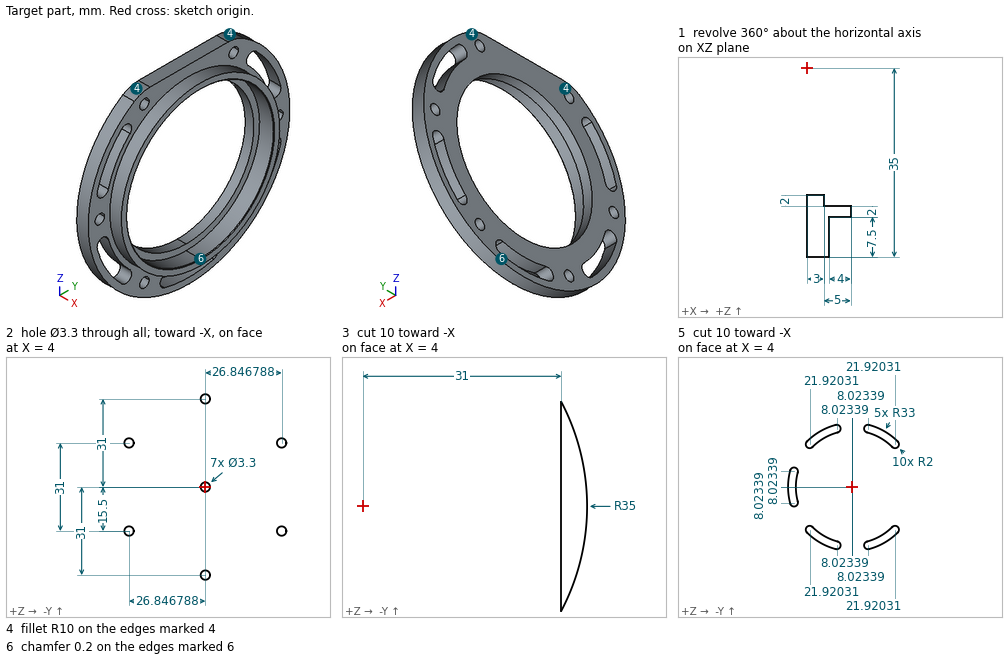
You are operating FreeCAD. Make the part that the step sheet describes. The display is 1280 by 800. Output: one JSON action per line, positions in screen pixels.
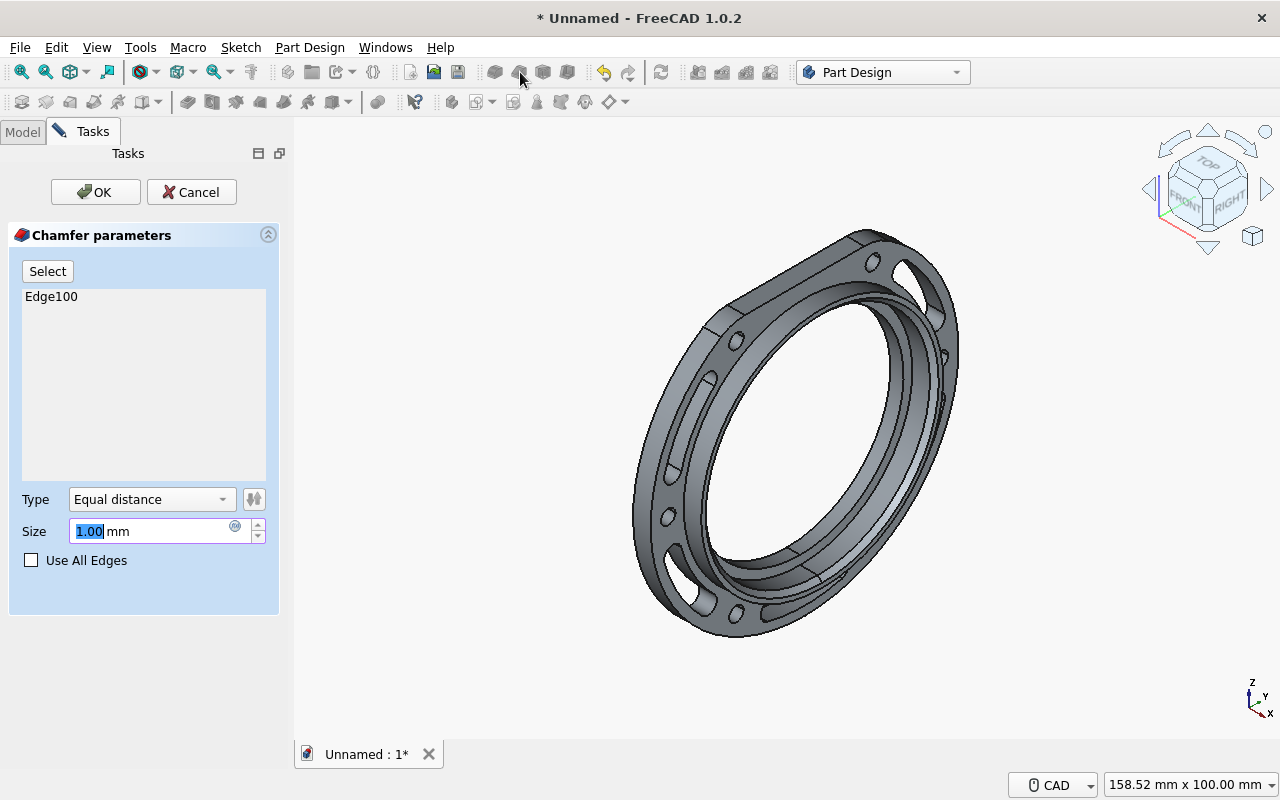
{"action": "type", "text": "0.2"}
{"action": "key", "text": "Tab"}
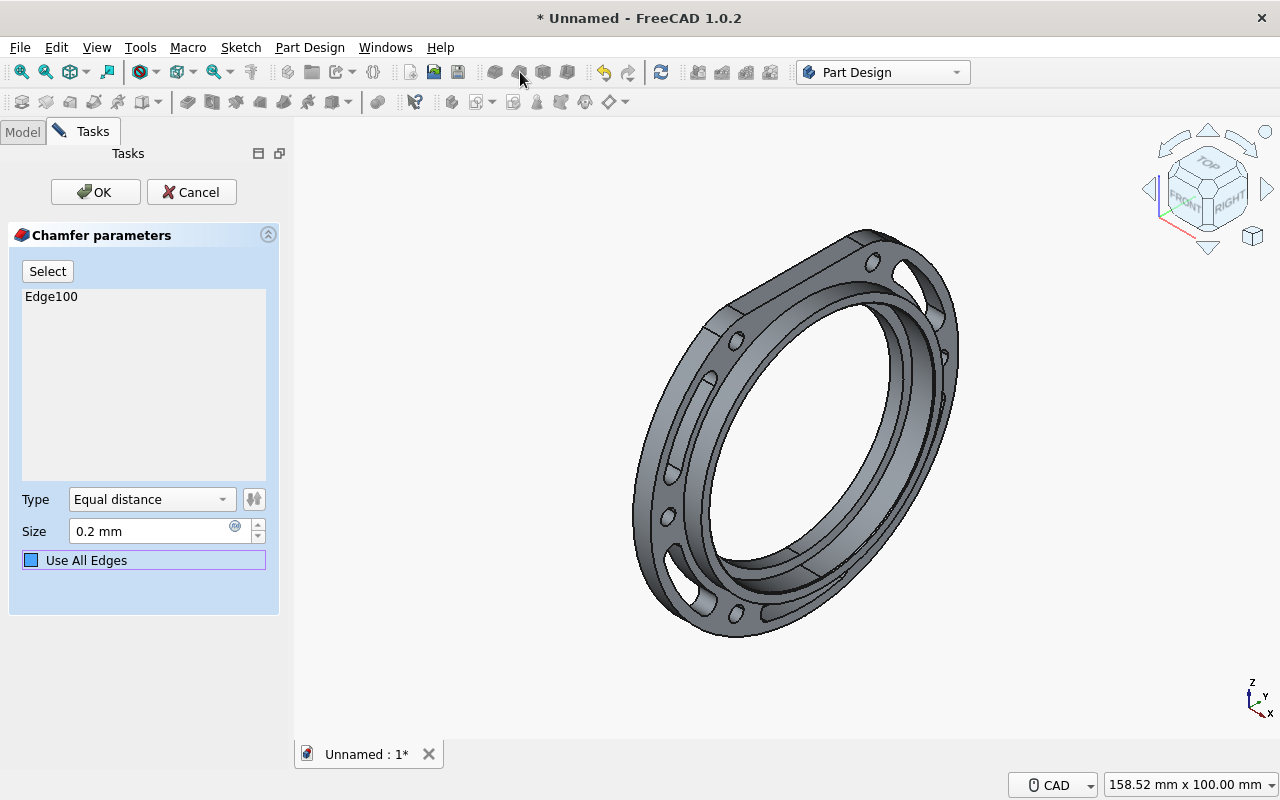
{"action": "left_click", "coordinate": [96, 192]}